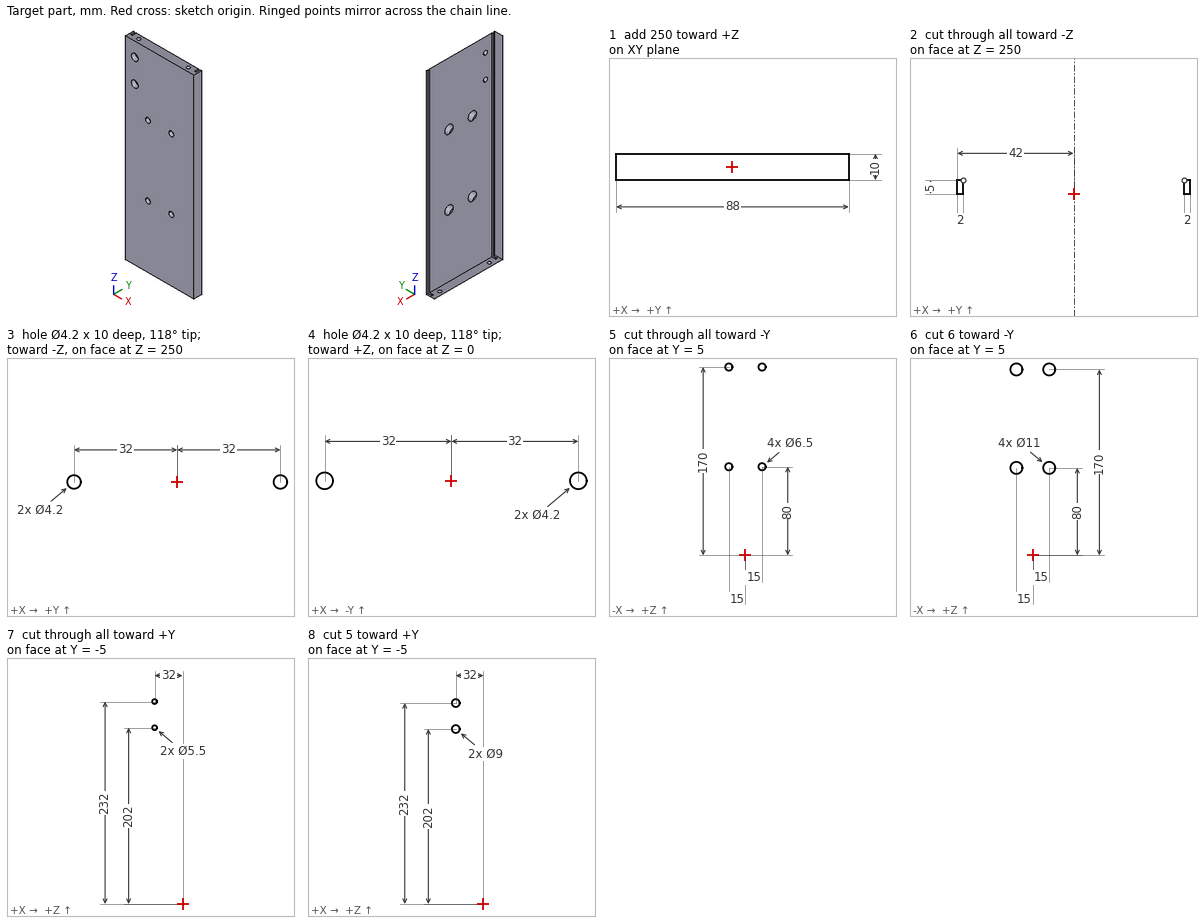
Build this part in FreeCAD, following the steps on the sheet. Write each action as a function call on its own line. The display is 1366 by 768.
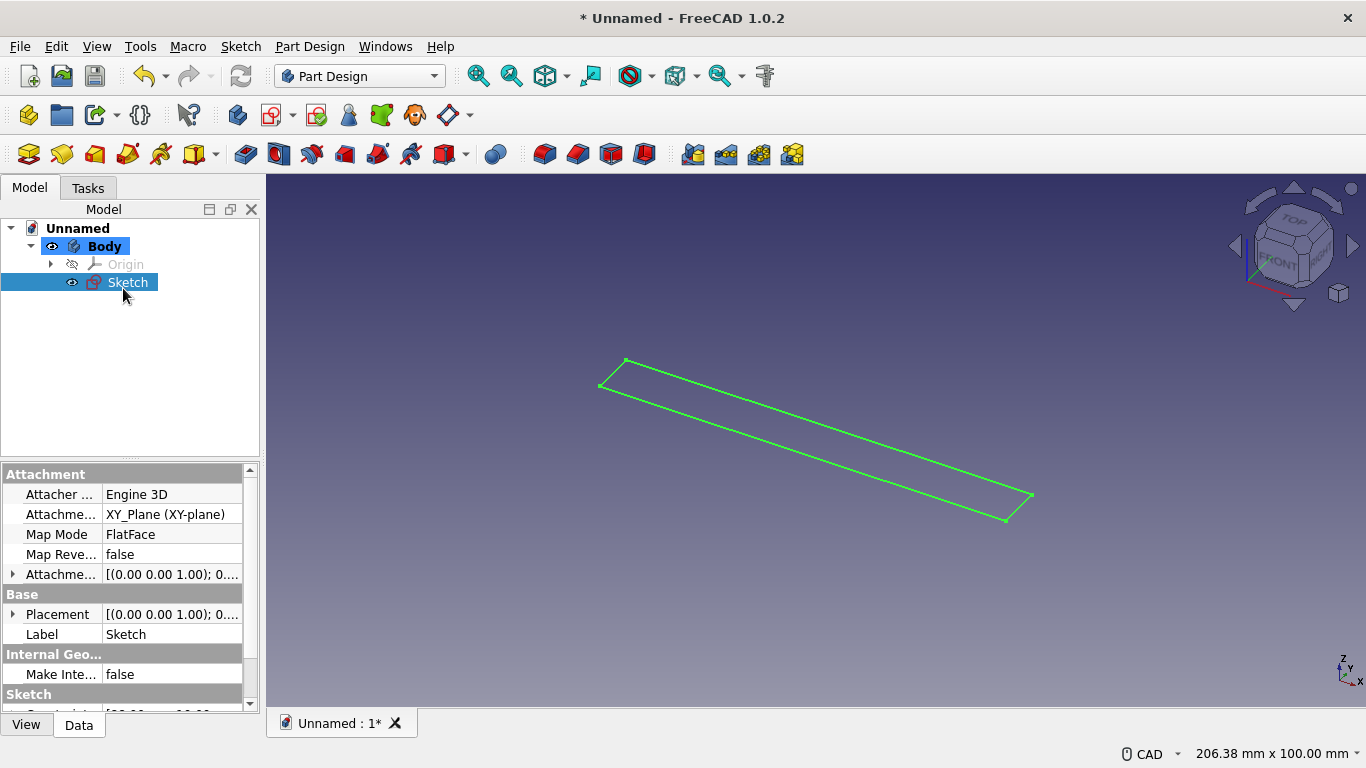
click(29, 154)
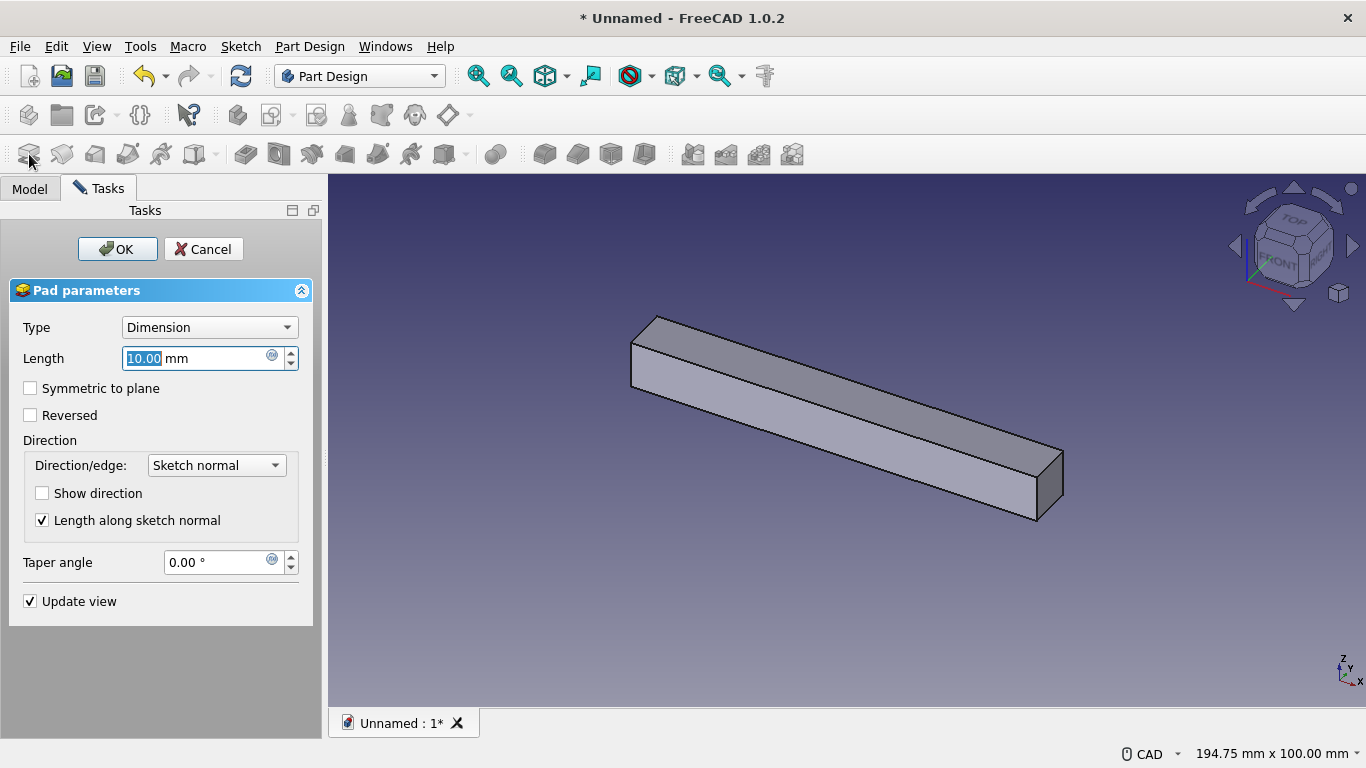
text(250)
key(Tab)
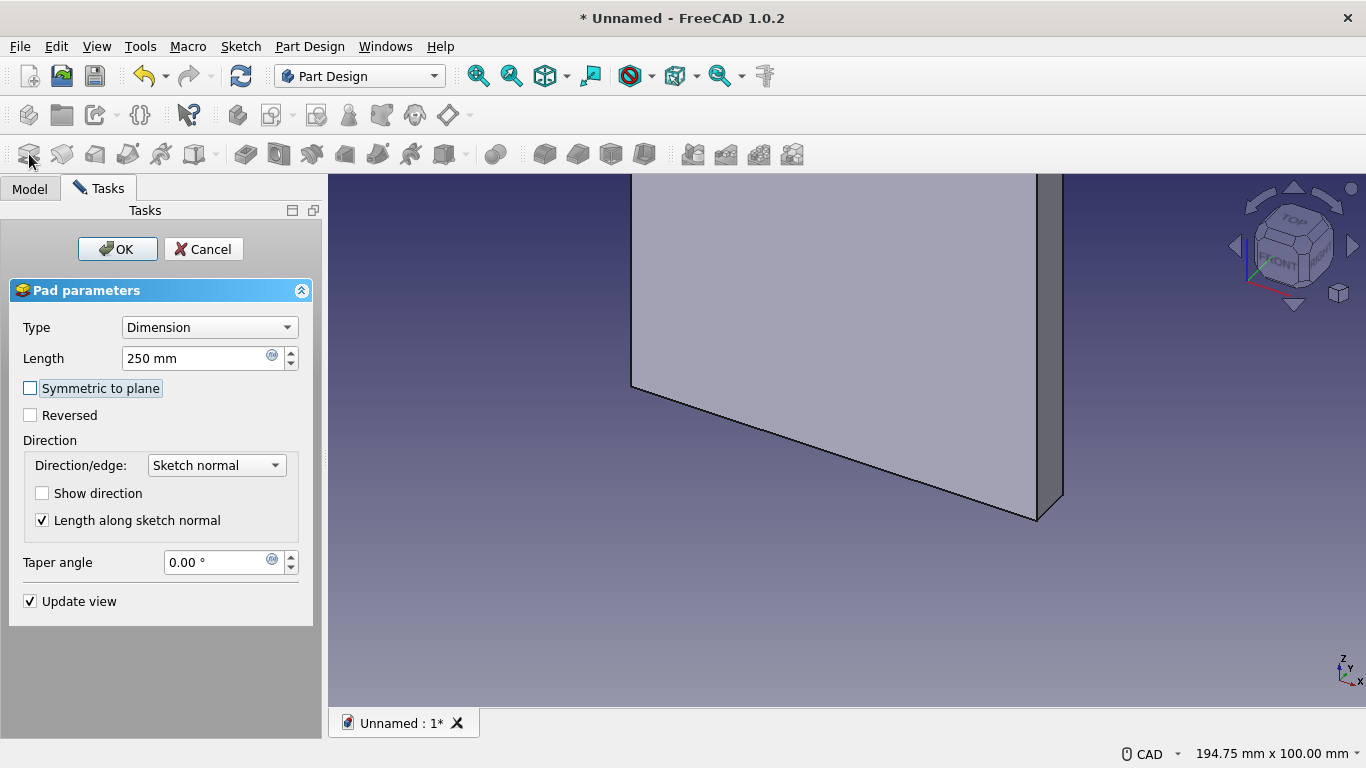
click(118, 249)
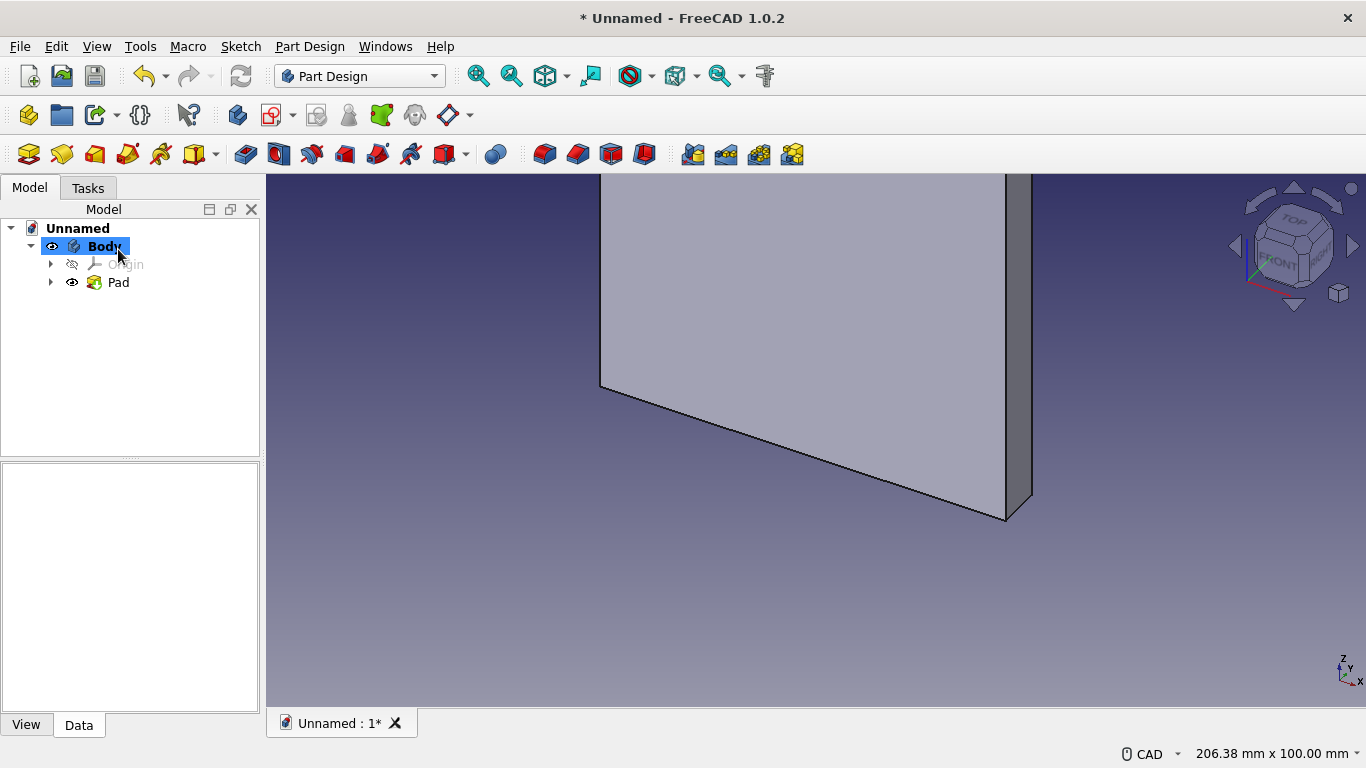
key(v)
key(f)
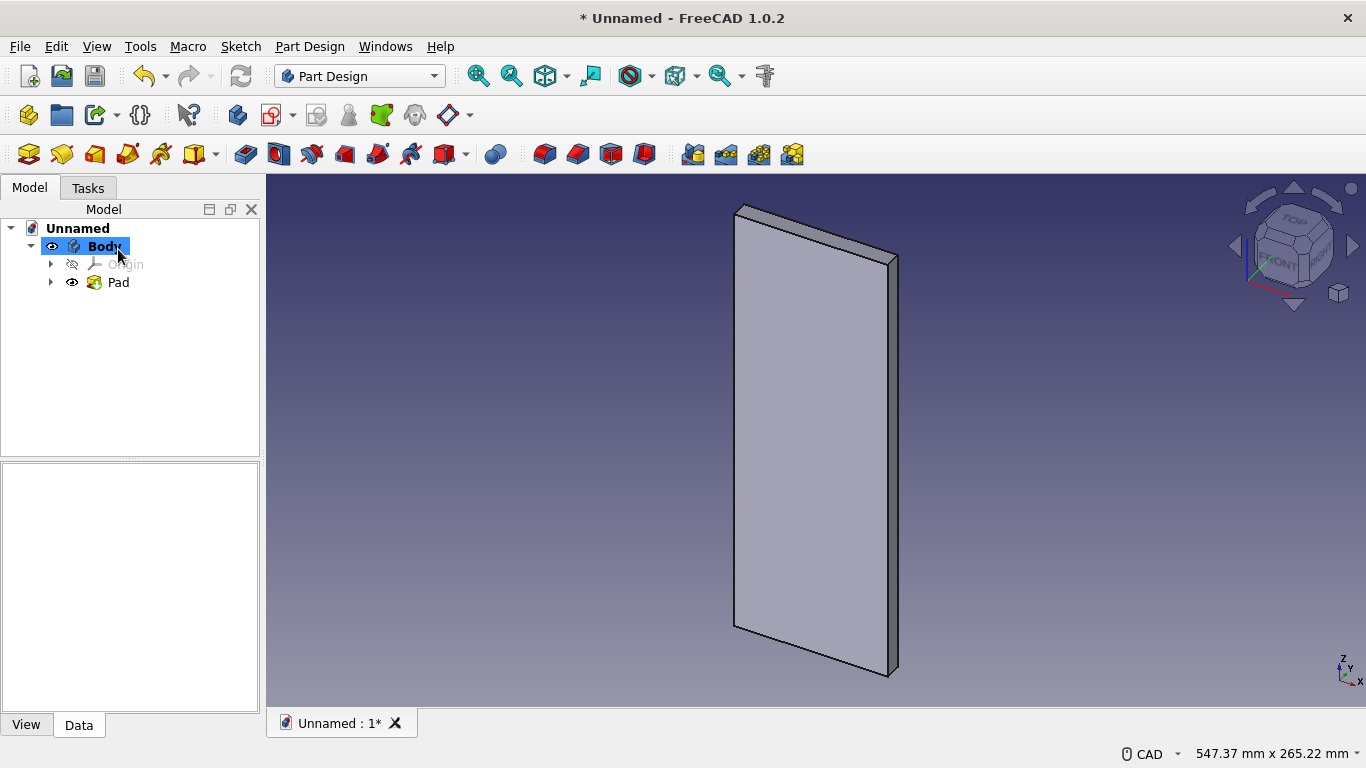
key(0)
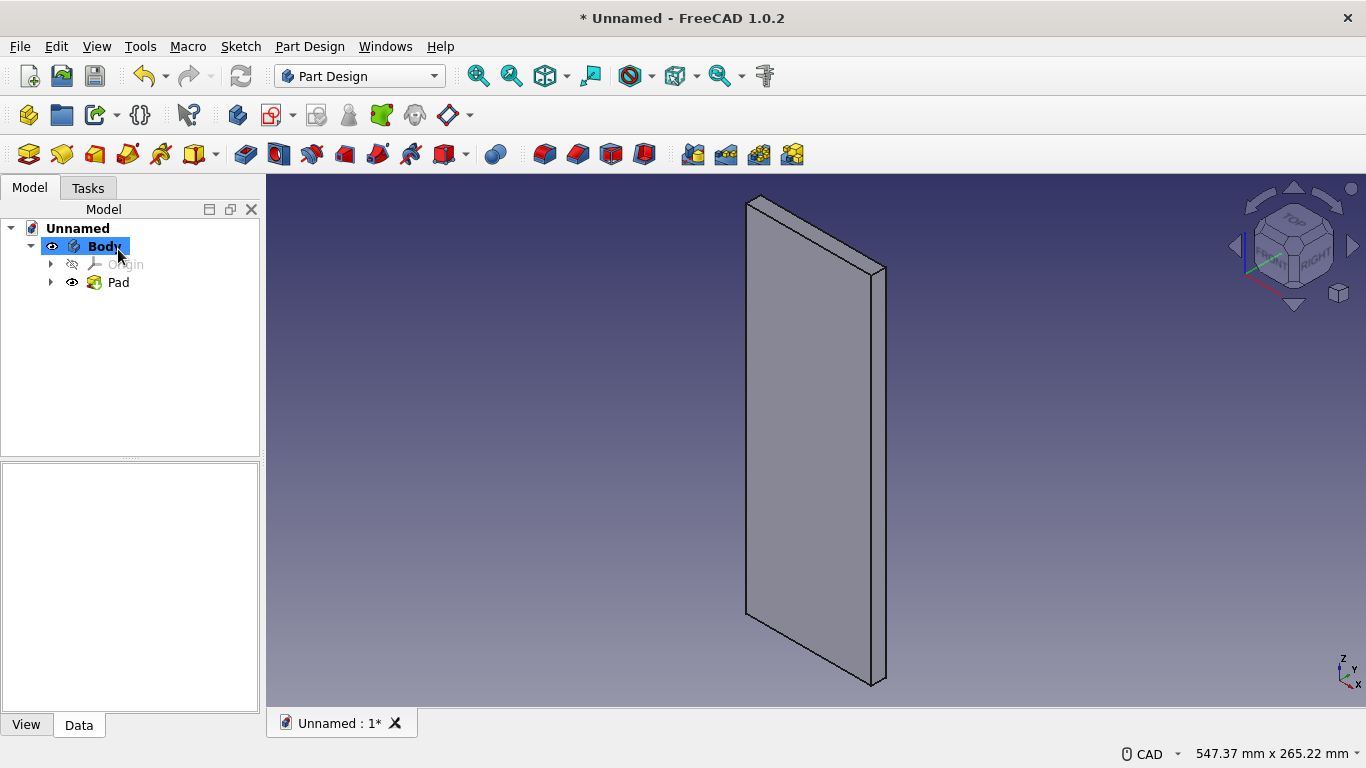
key(2)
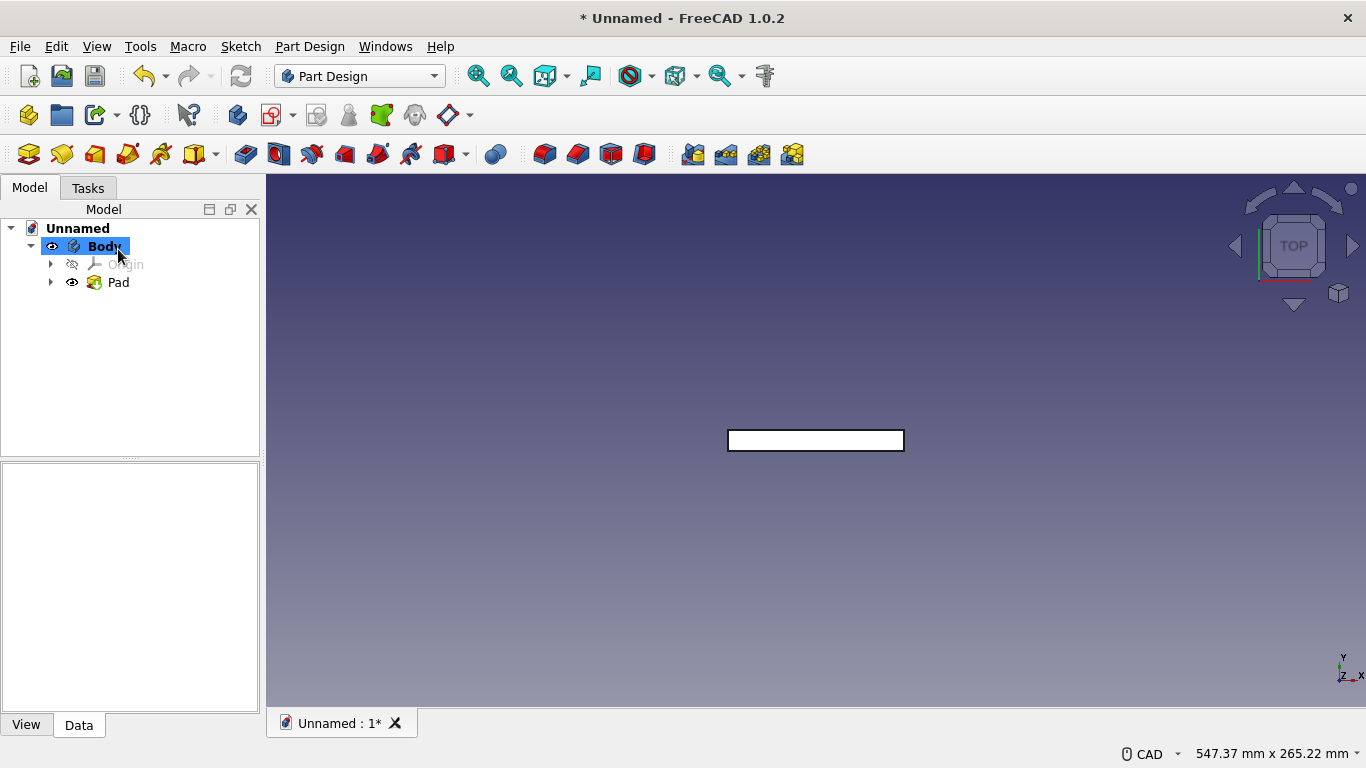
click(479, 76)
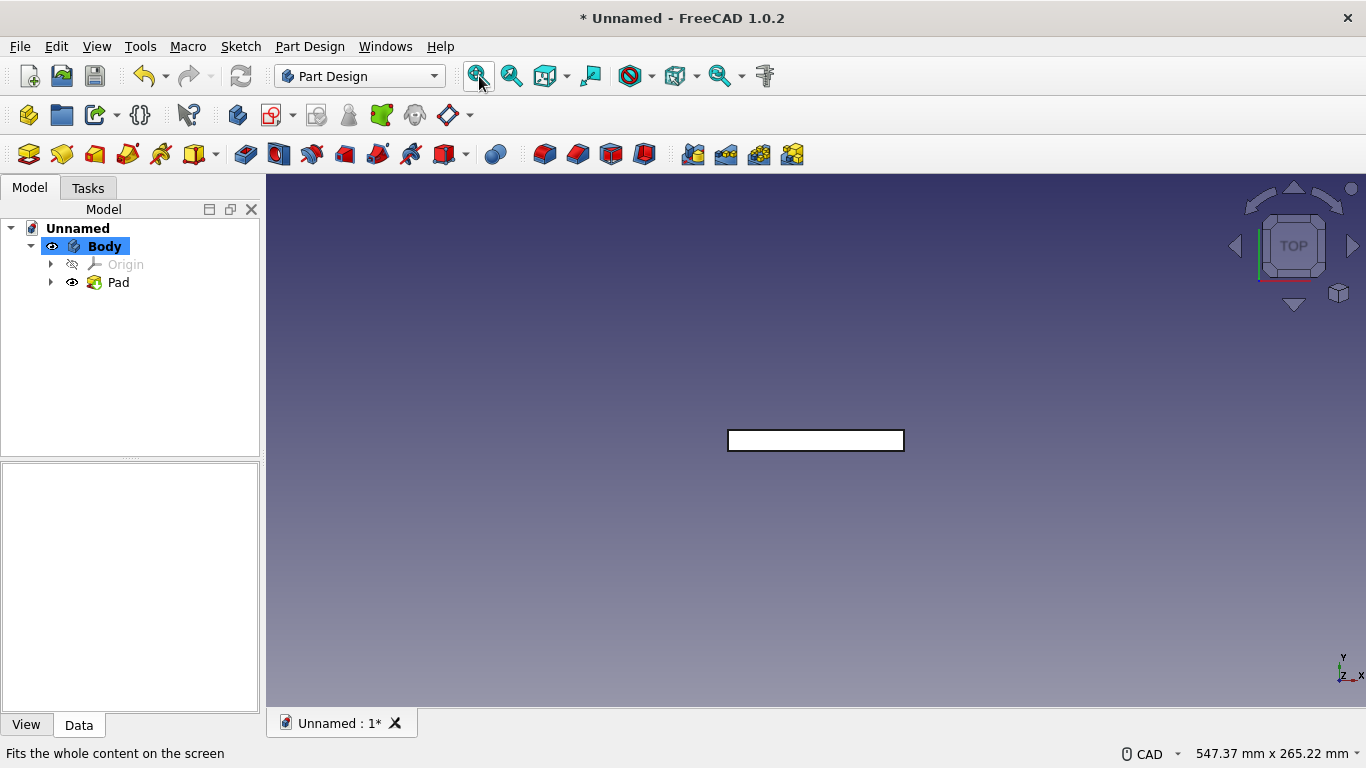
click(892, 439)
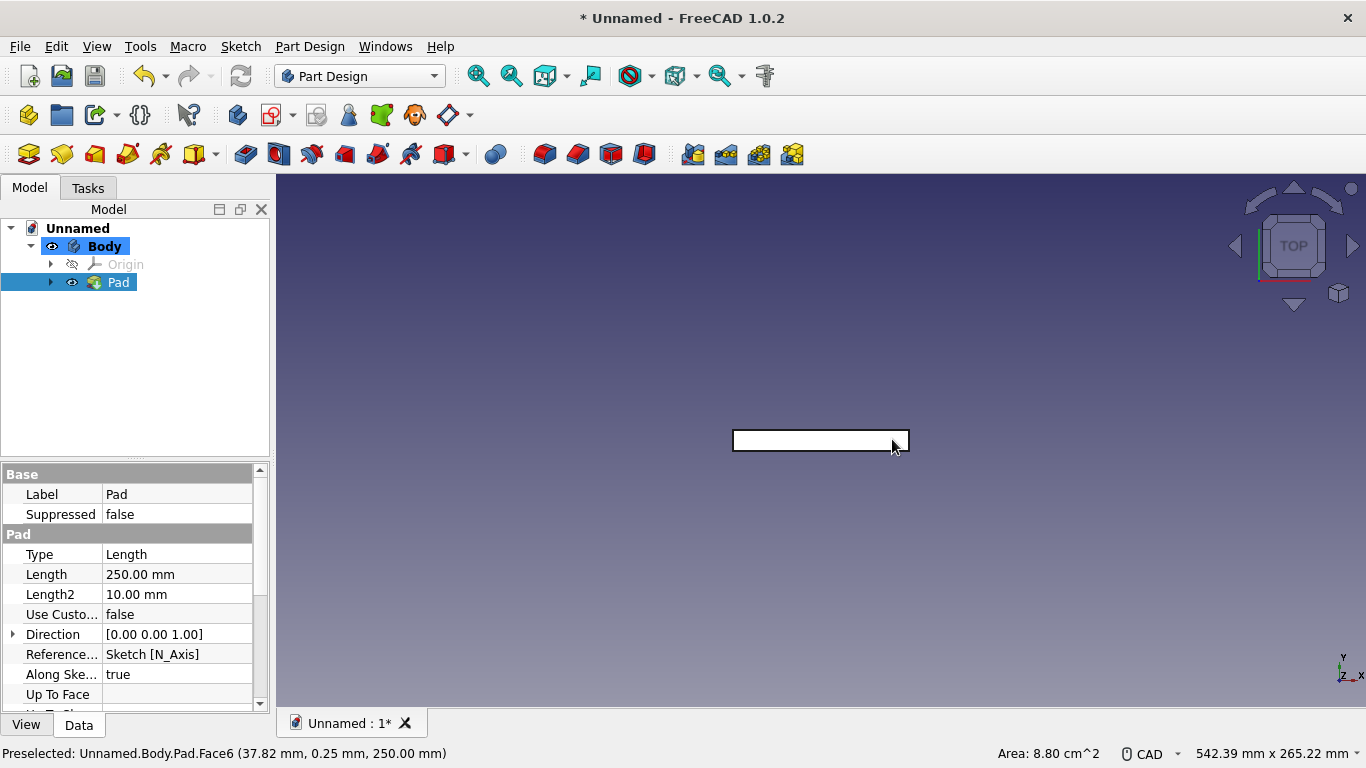
click(270, 116)